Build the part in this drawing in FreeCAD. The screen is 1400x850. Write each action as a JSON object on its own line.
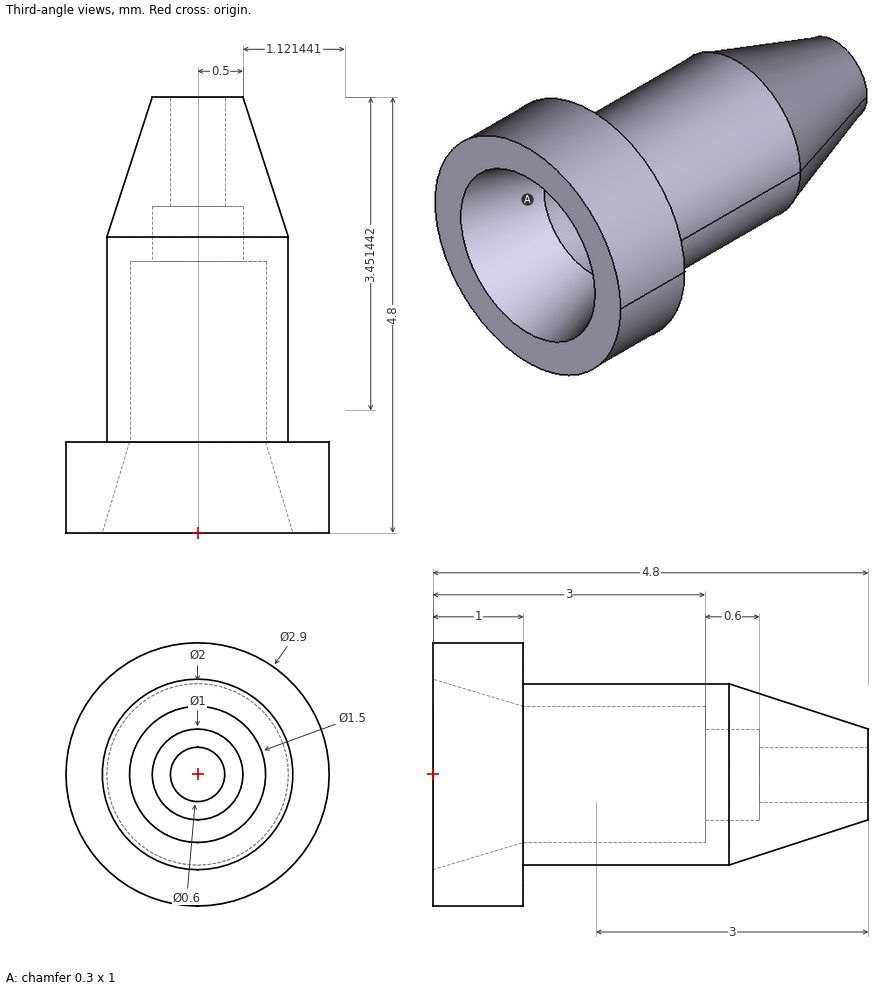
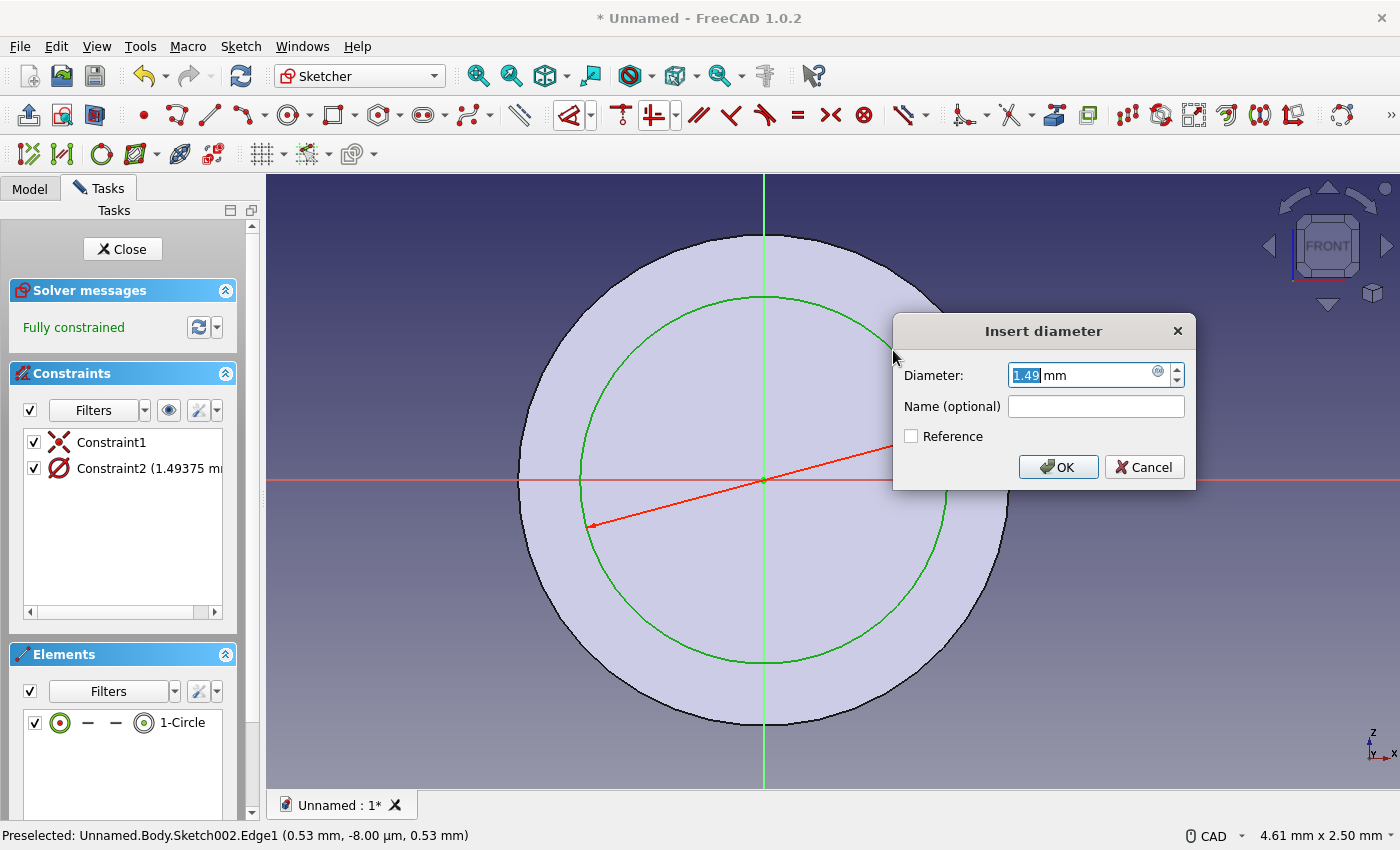
{"action": "type", "text": "1.5"}
{"action": "key", "text": "Return"}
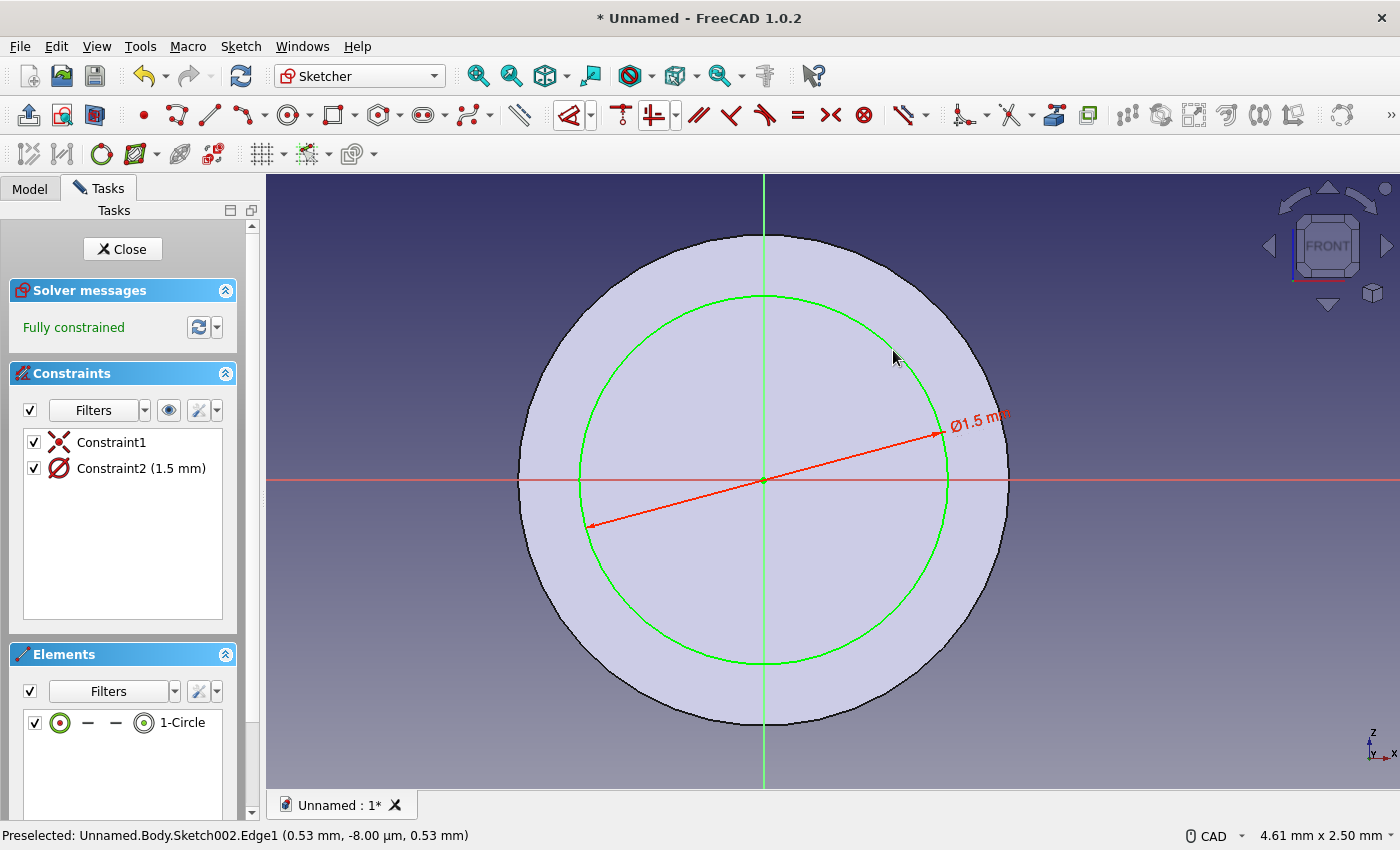
{"action": "left_click", "coordinate": [123, 249]}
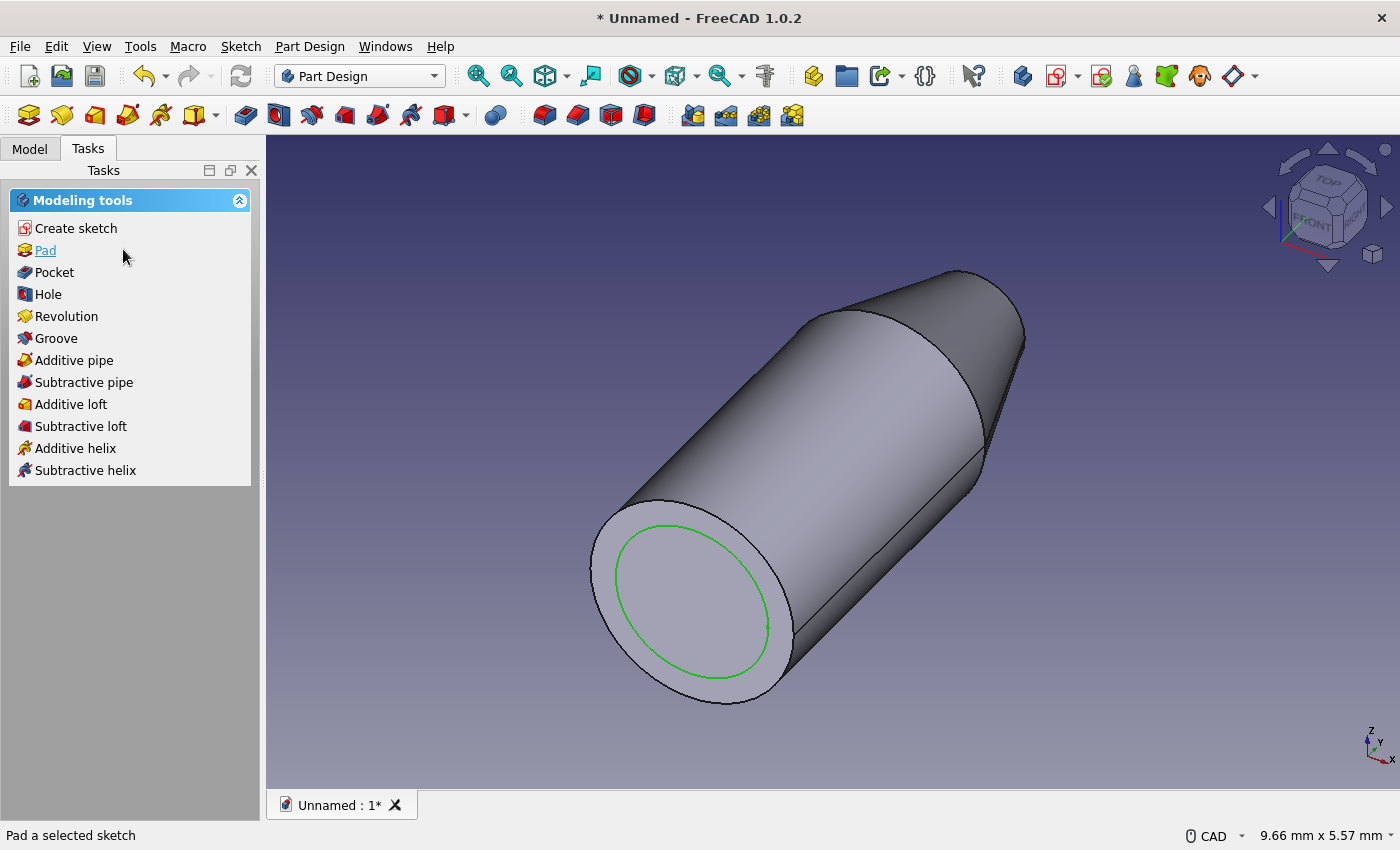
{"action": "left_click", "coordinate": [246, 116]}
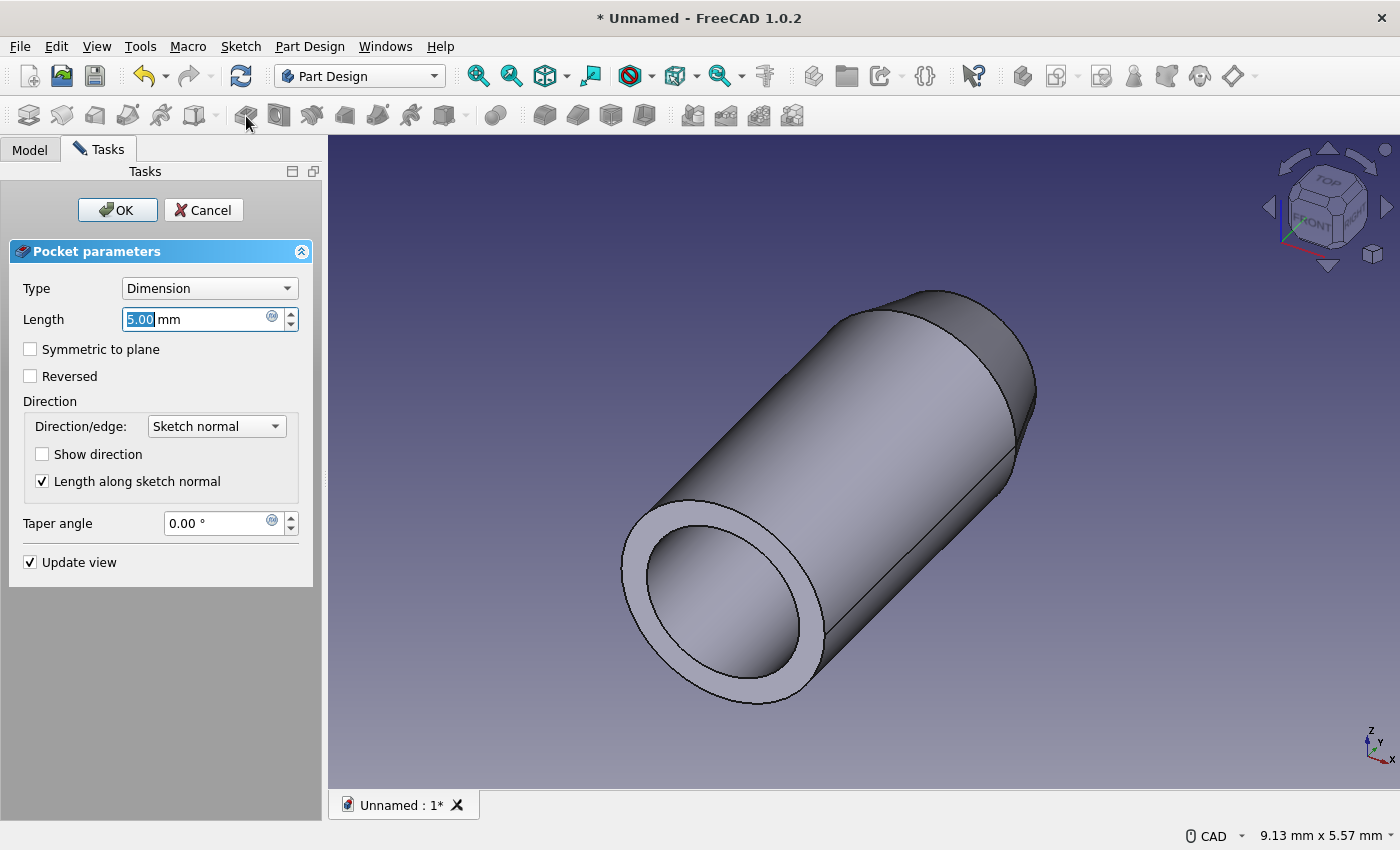
{"action": "type", "text": "3"}
{"action": "key", "text": "Tab"}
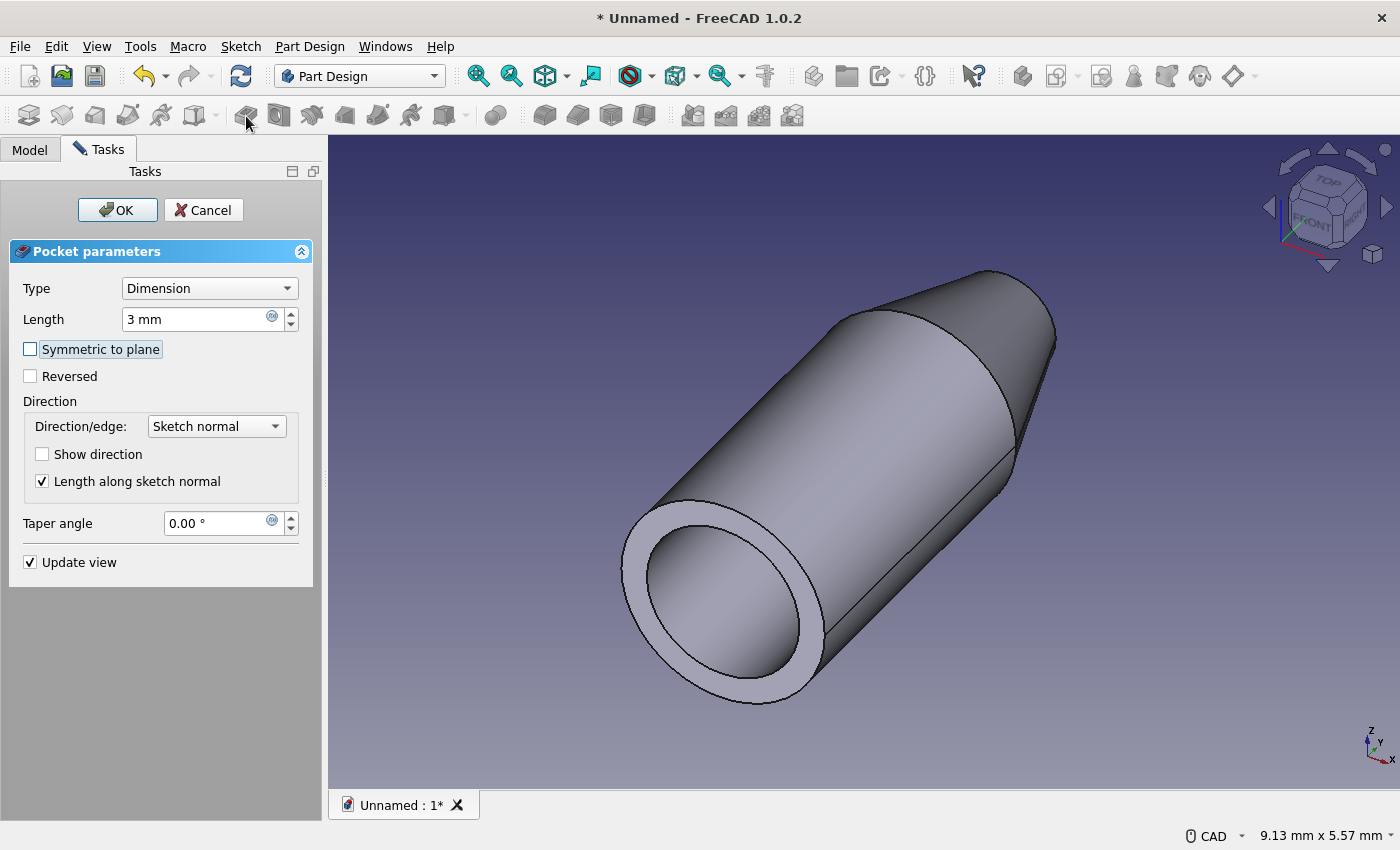
{"action": "left_click", "coordinate": [118, 210]}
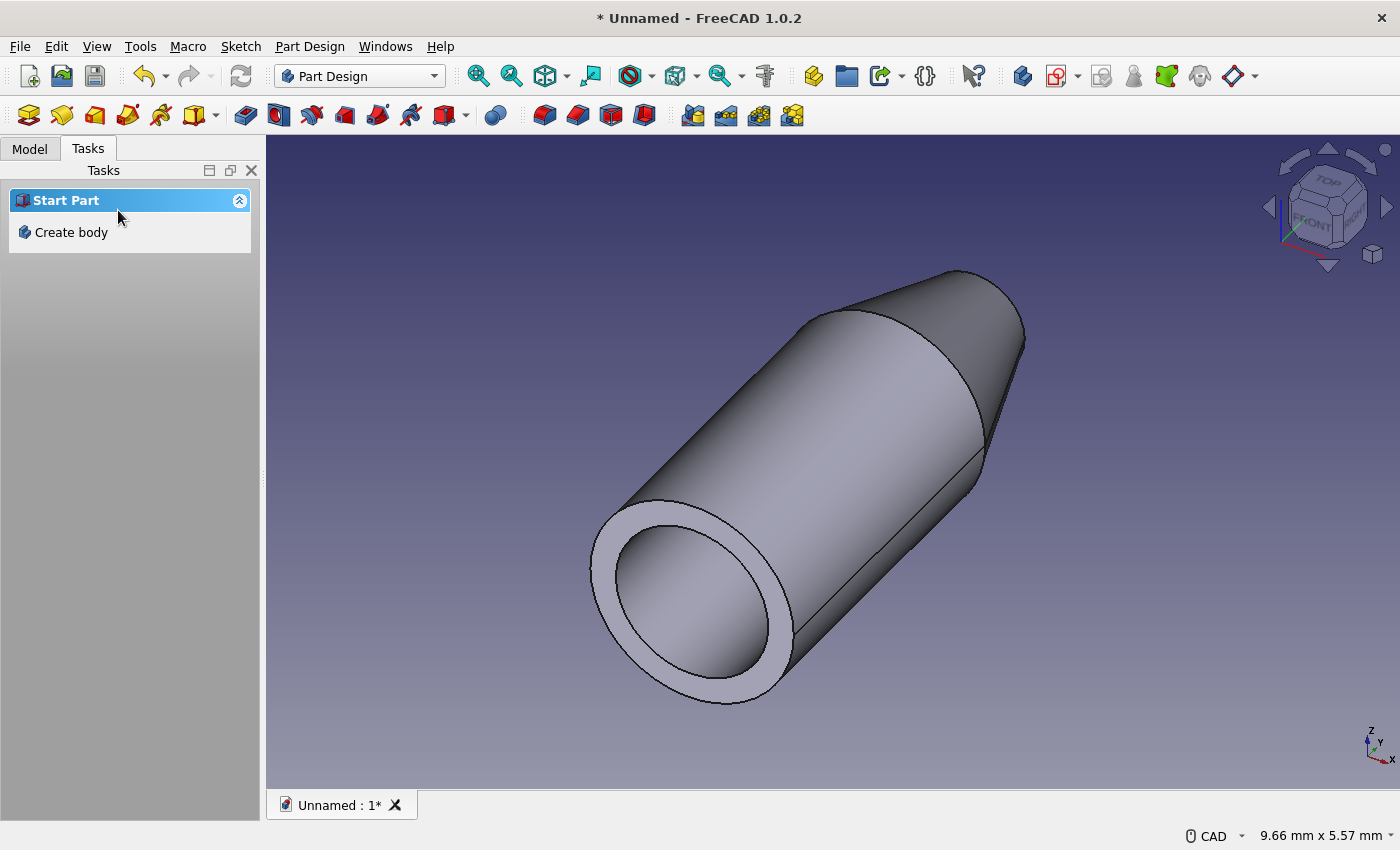
{"action": "key", "text": "4"}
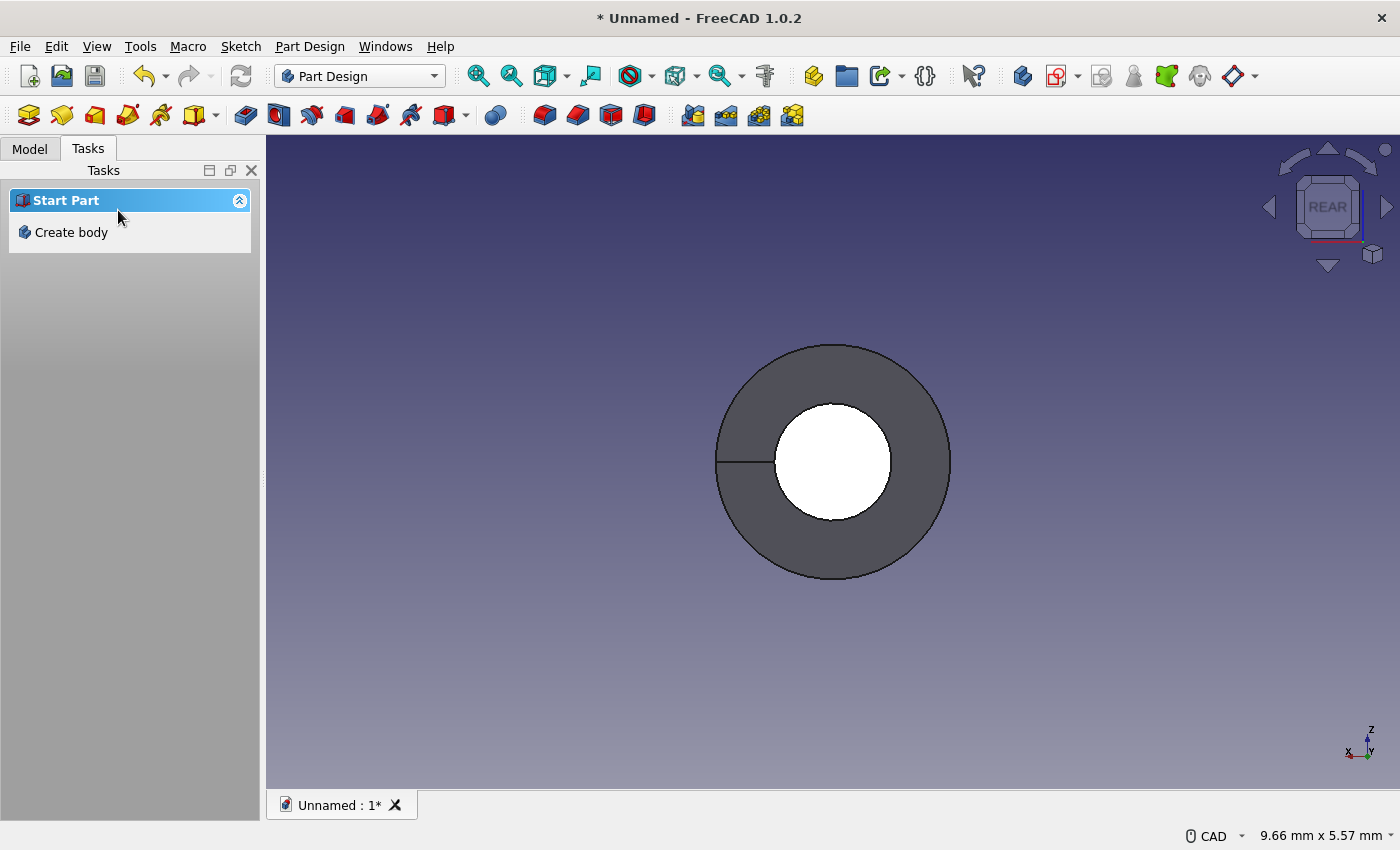
{"action": "left_click", "coordinate": [479, 76]}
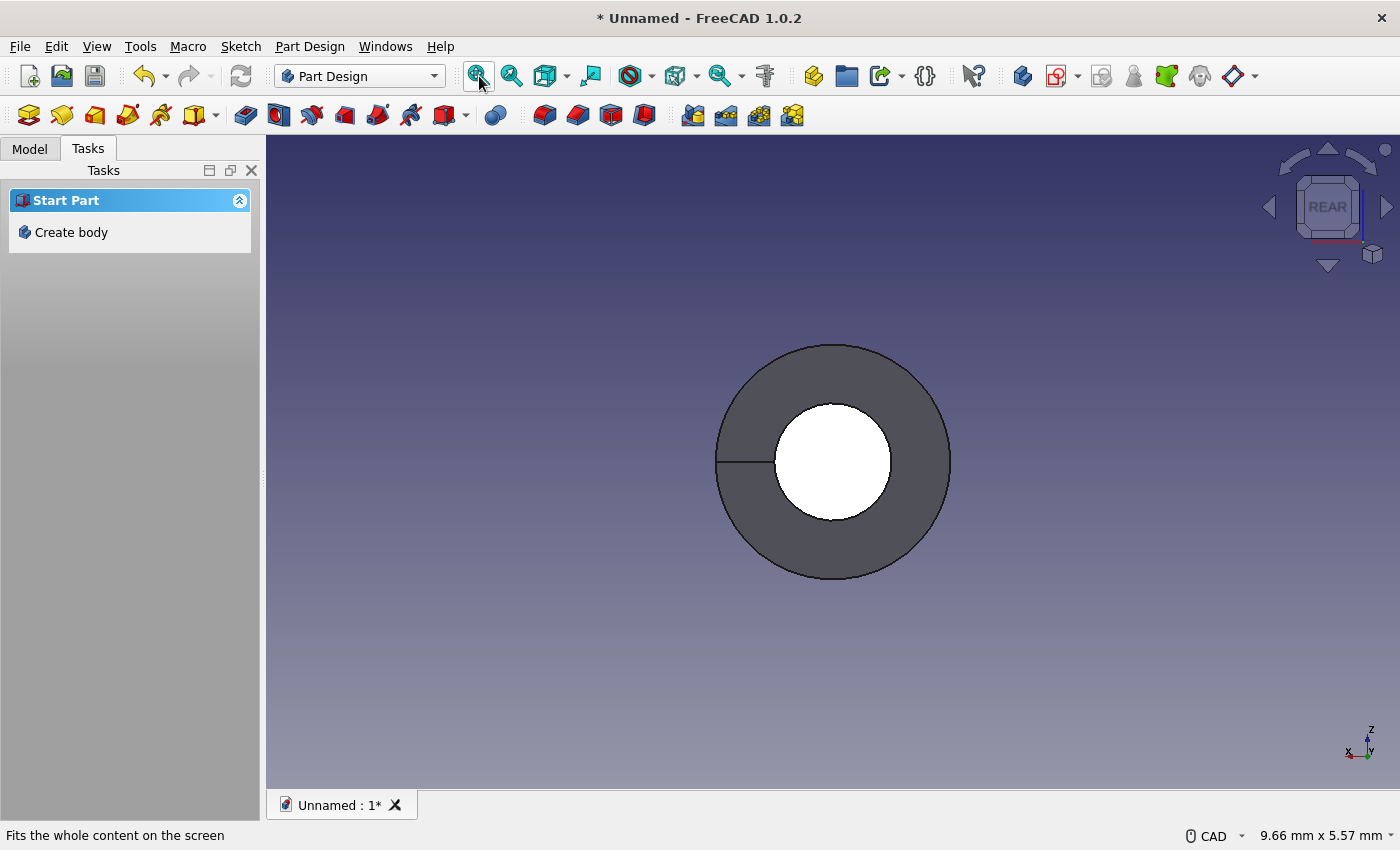
{"action": "left_click", "coordinate": [833, 461]}